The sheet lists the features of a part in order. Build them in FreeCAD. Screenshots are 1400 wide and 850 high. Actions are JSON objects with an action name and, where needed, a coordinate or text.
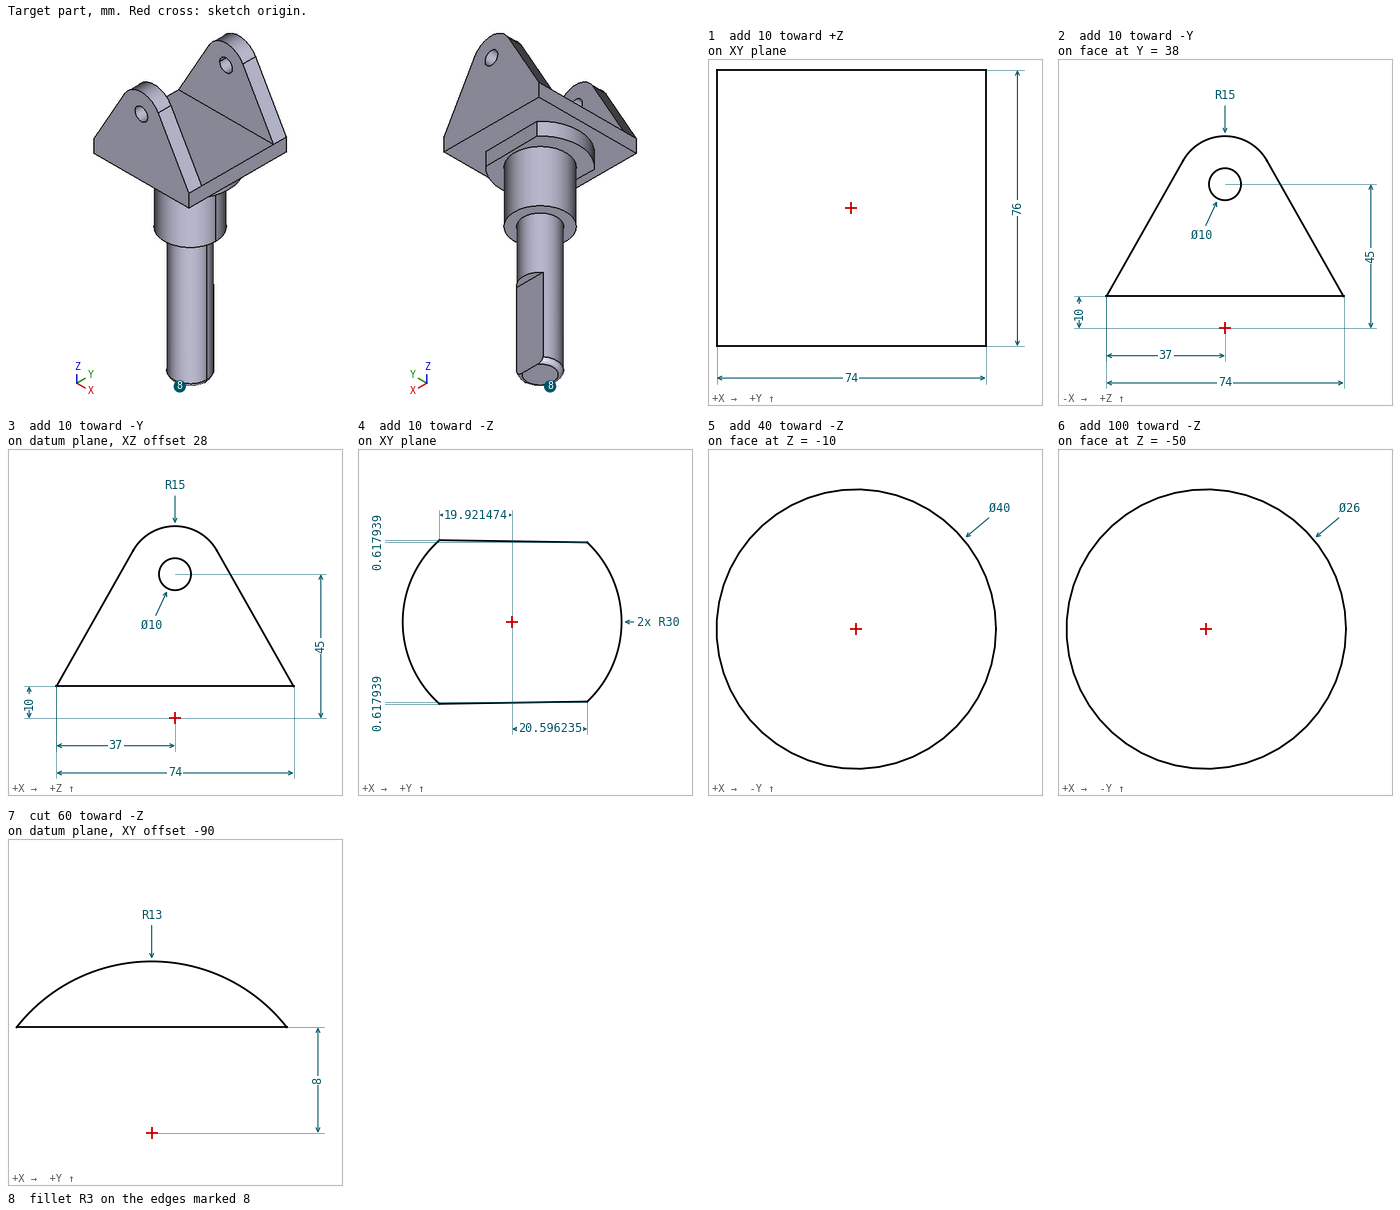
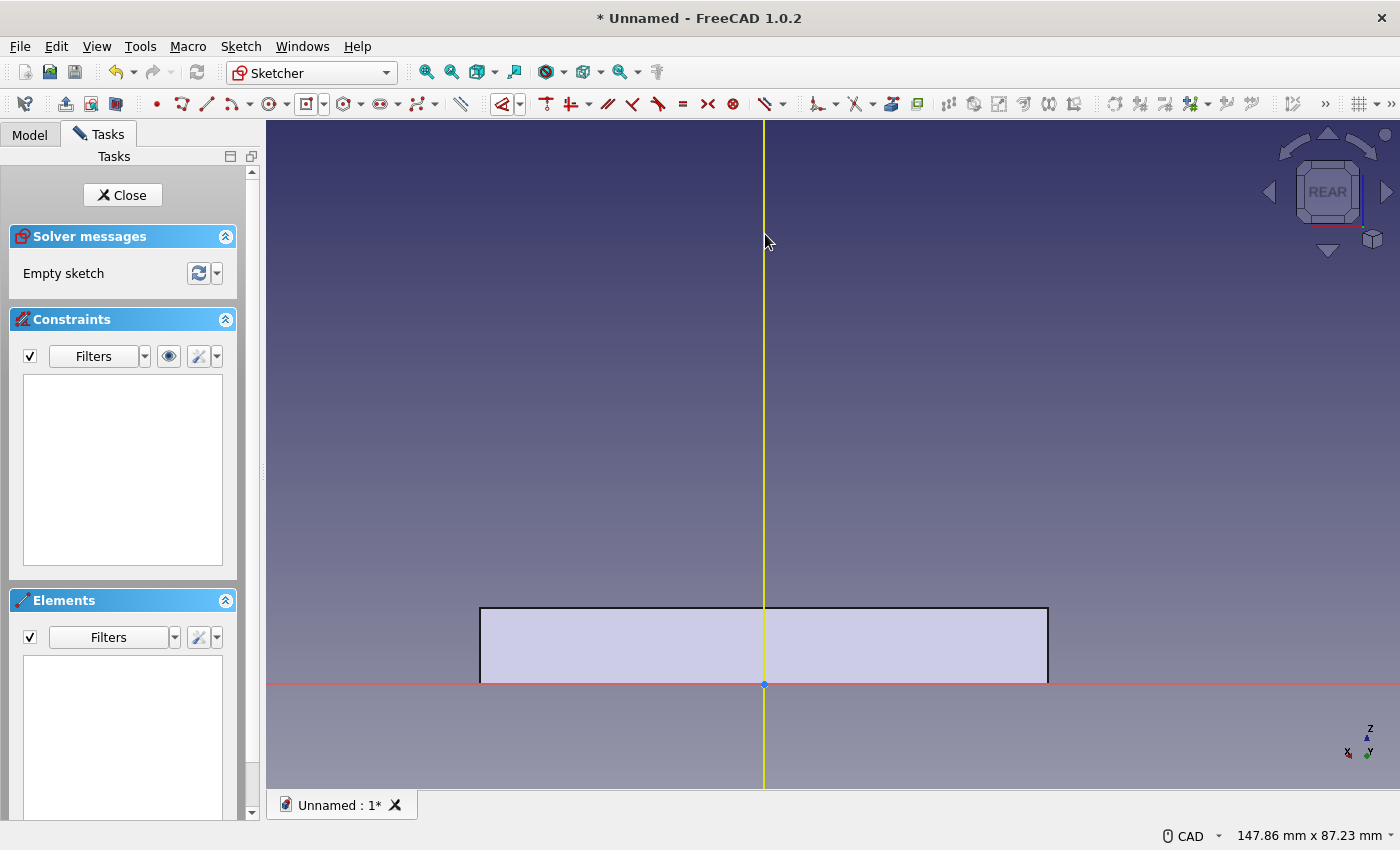
{"action": "left_click", "coordinate": [182, 104]}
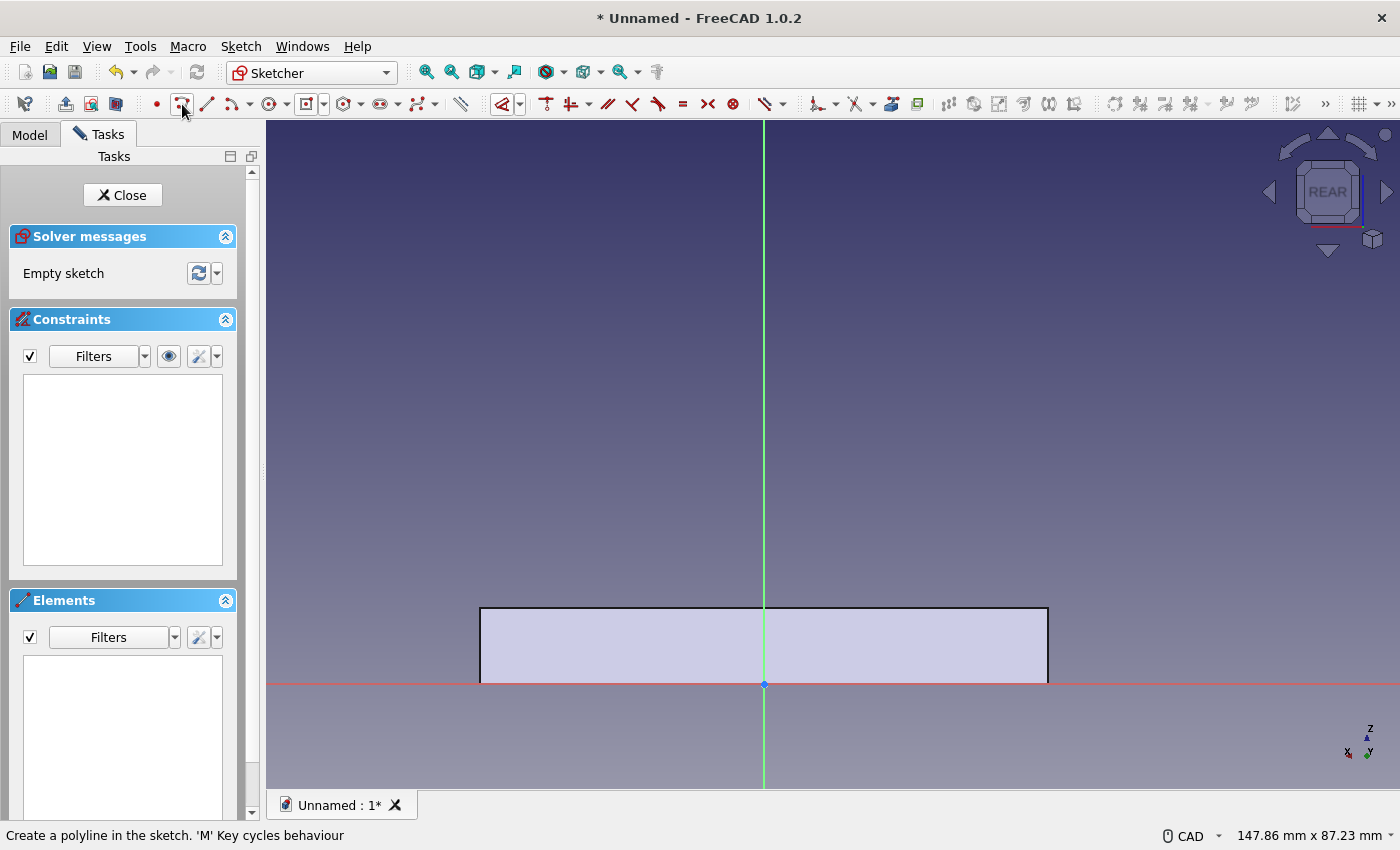
{"action": "left_click", "coordinate": [664, 283]}
{"action": "left_click", "coordinate": [480, 608]}
{"action": "left_click", "coordinate": [1048, 608]}
{"action": "left_click", "coordinate": [864, 283]}
{"action": "right_click", "coordinate": [864, 283]}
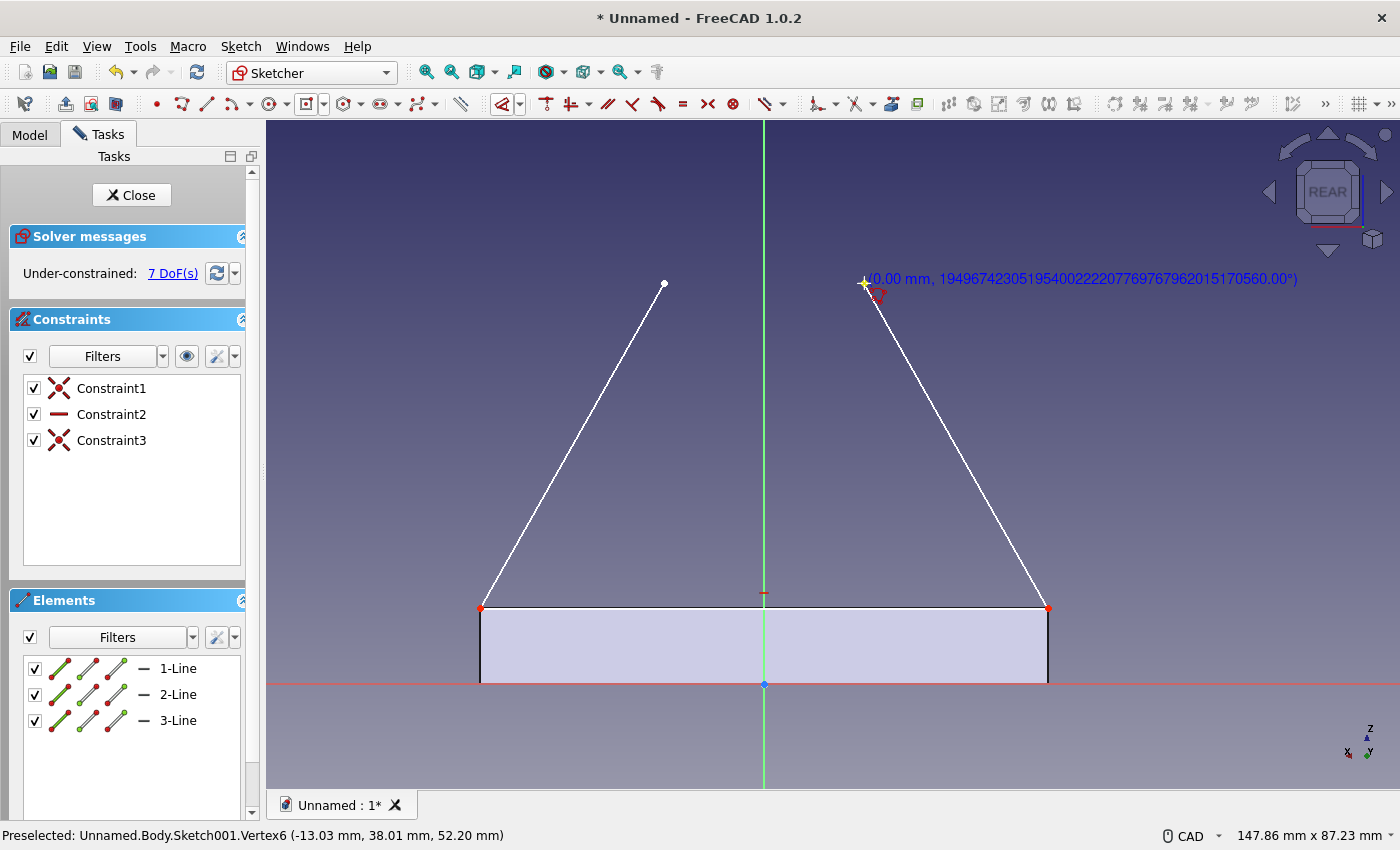
{"action": "key", "text": "g 3 a"}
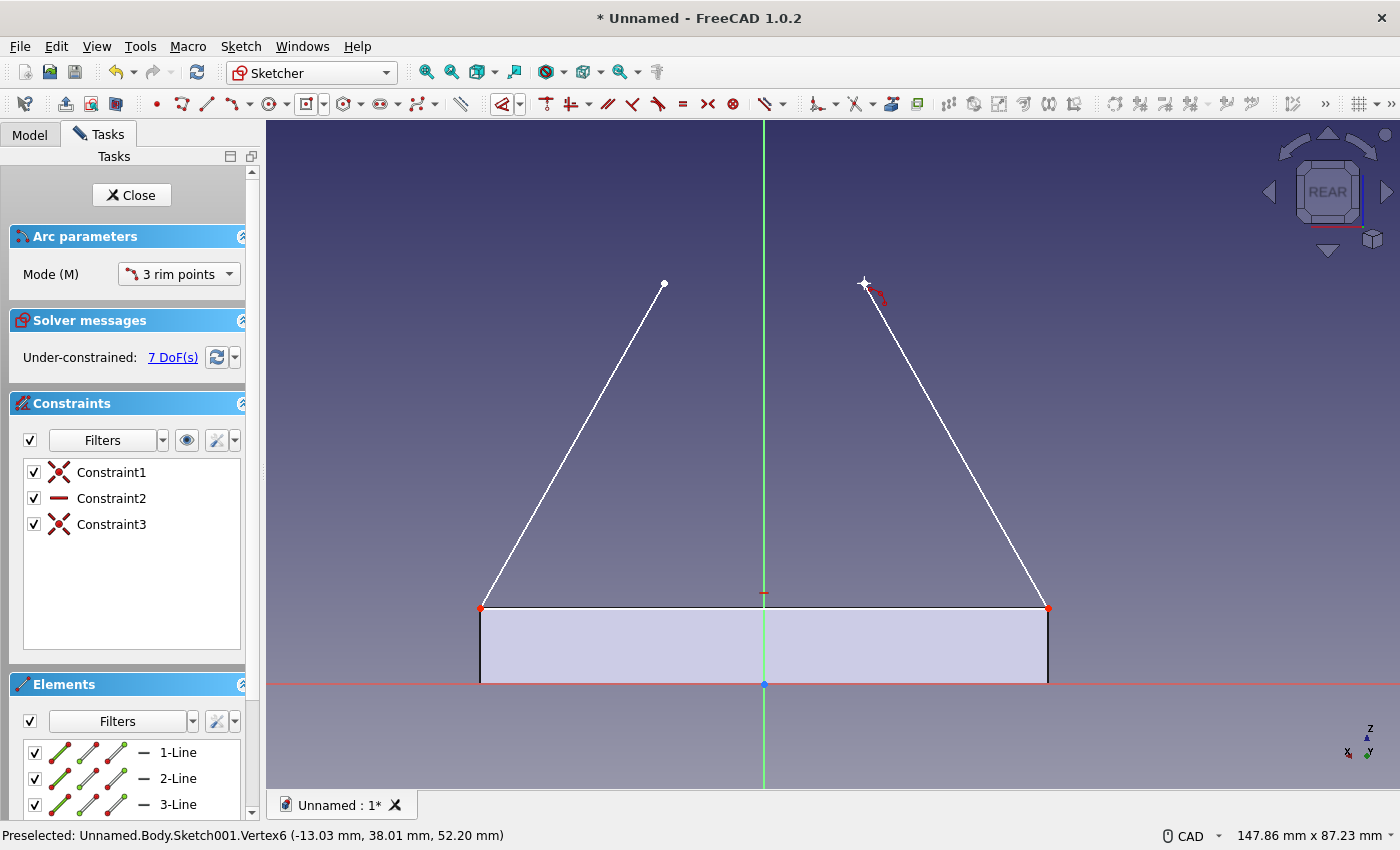
{"action": "left_click", "coordinate": [864, 284]}
{"action": "left_click", "coordinate": [664, 284]}
{"action": "left_click", "coordinate": [788, 227]}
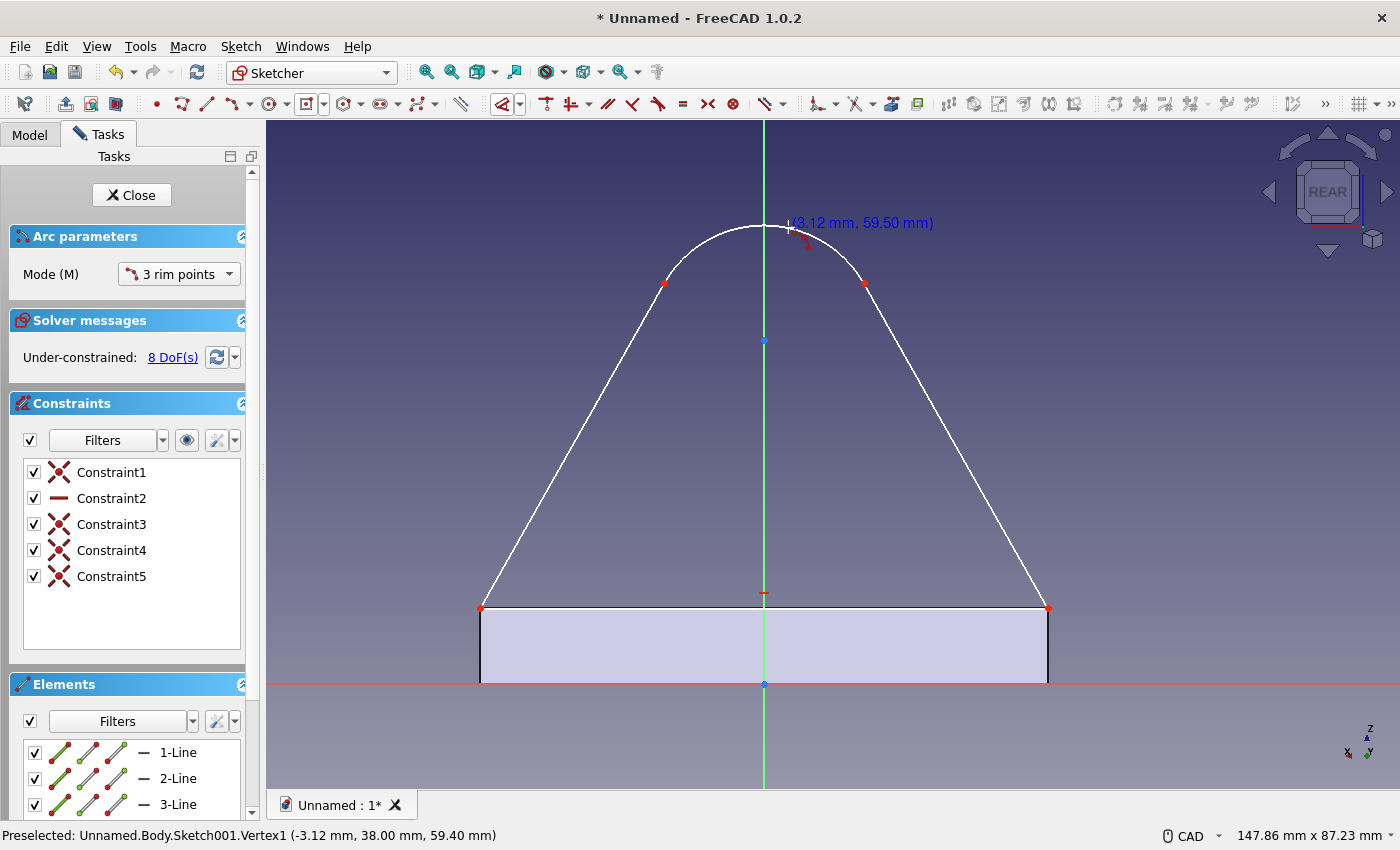
{"action": "left_click", "coordinate": [268, 104]}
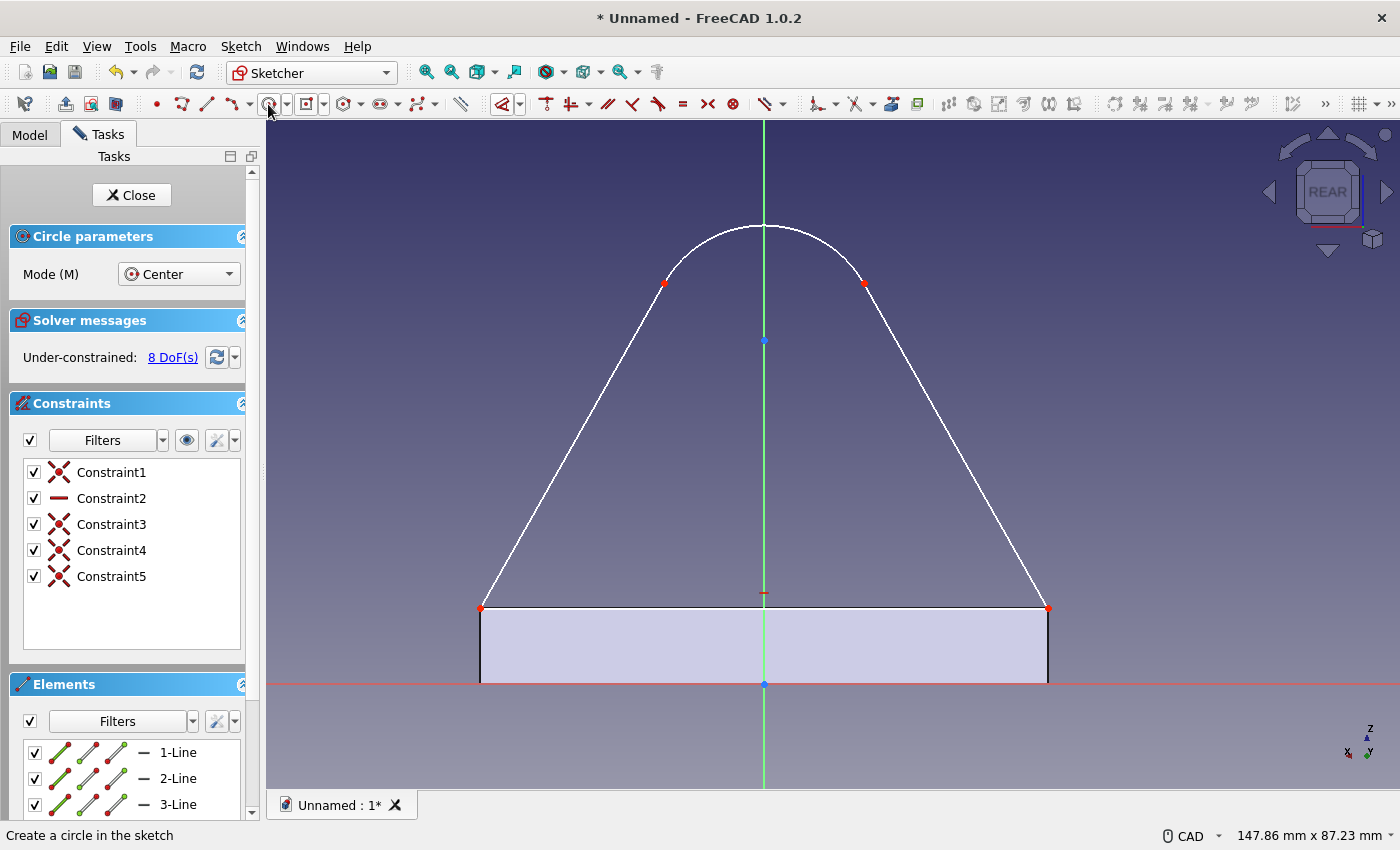
{"action": "left_click", "coordinate": [764, 339]}
{"action": "left_click", "coordinate": [791, 312]}
{"action": "key", "text": "Escape"}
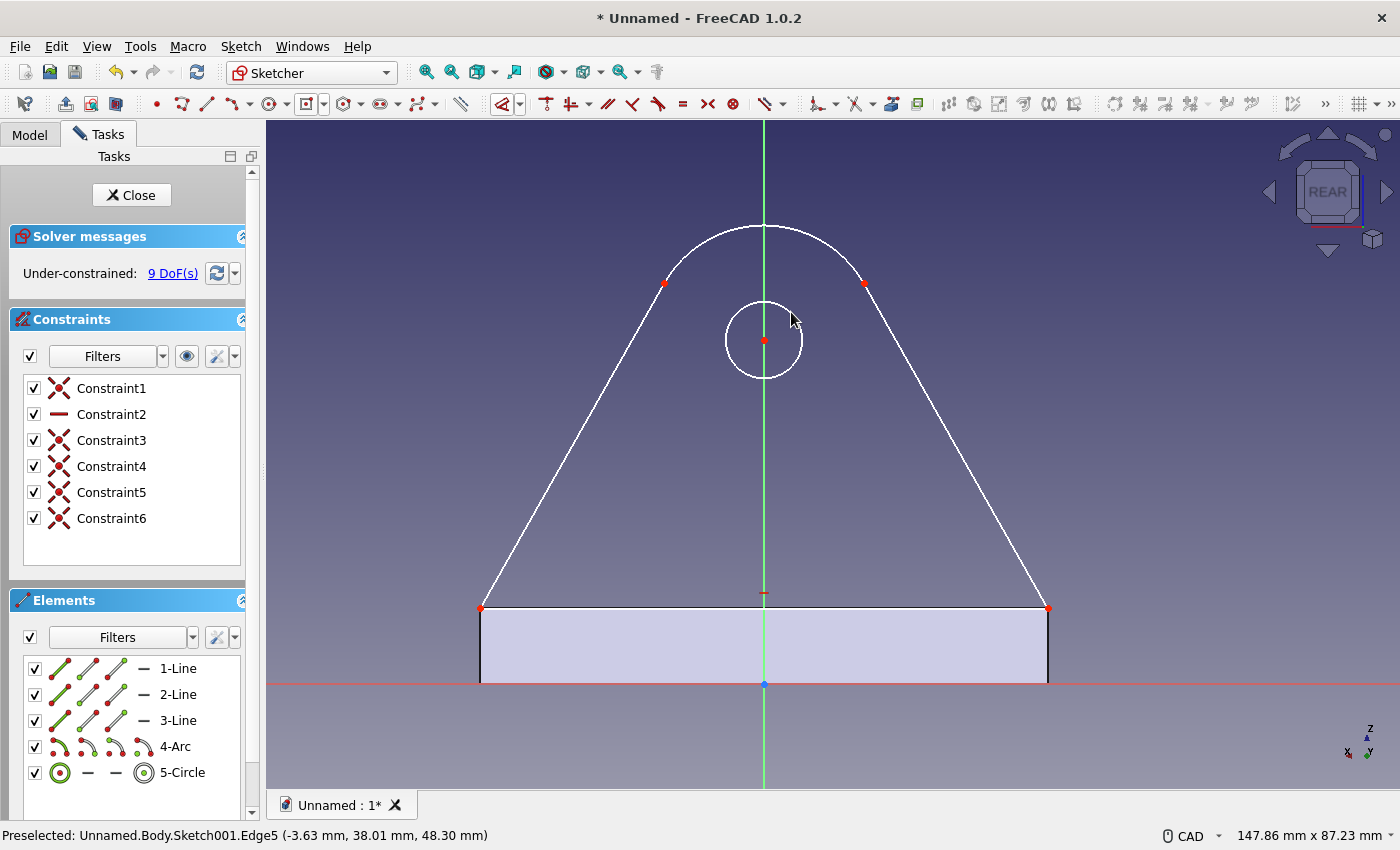
{"action": "left_click", "coordinate": [609, 381]}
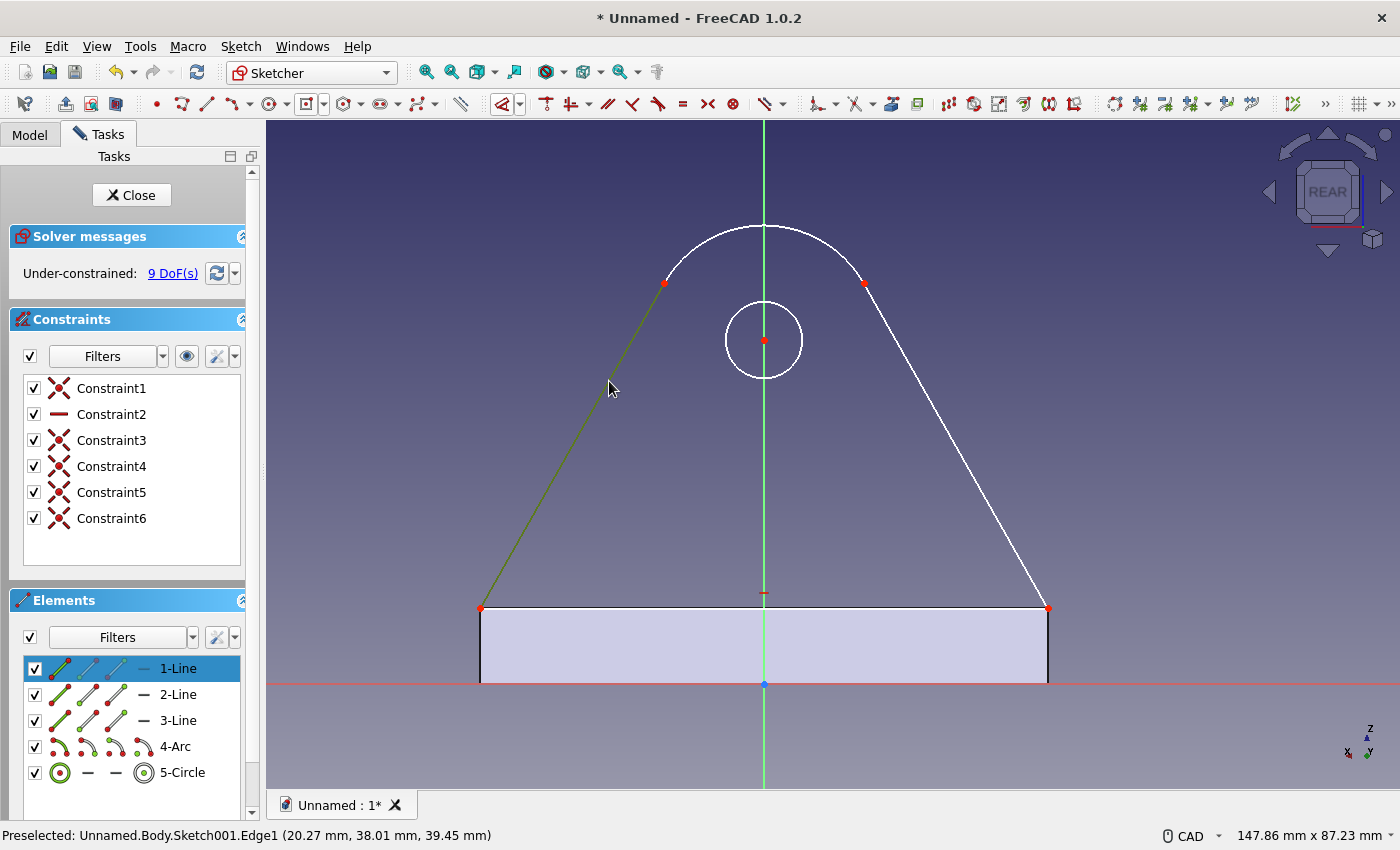
{"action": "left_click", "coordinate": [811, 236]}